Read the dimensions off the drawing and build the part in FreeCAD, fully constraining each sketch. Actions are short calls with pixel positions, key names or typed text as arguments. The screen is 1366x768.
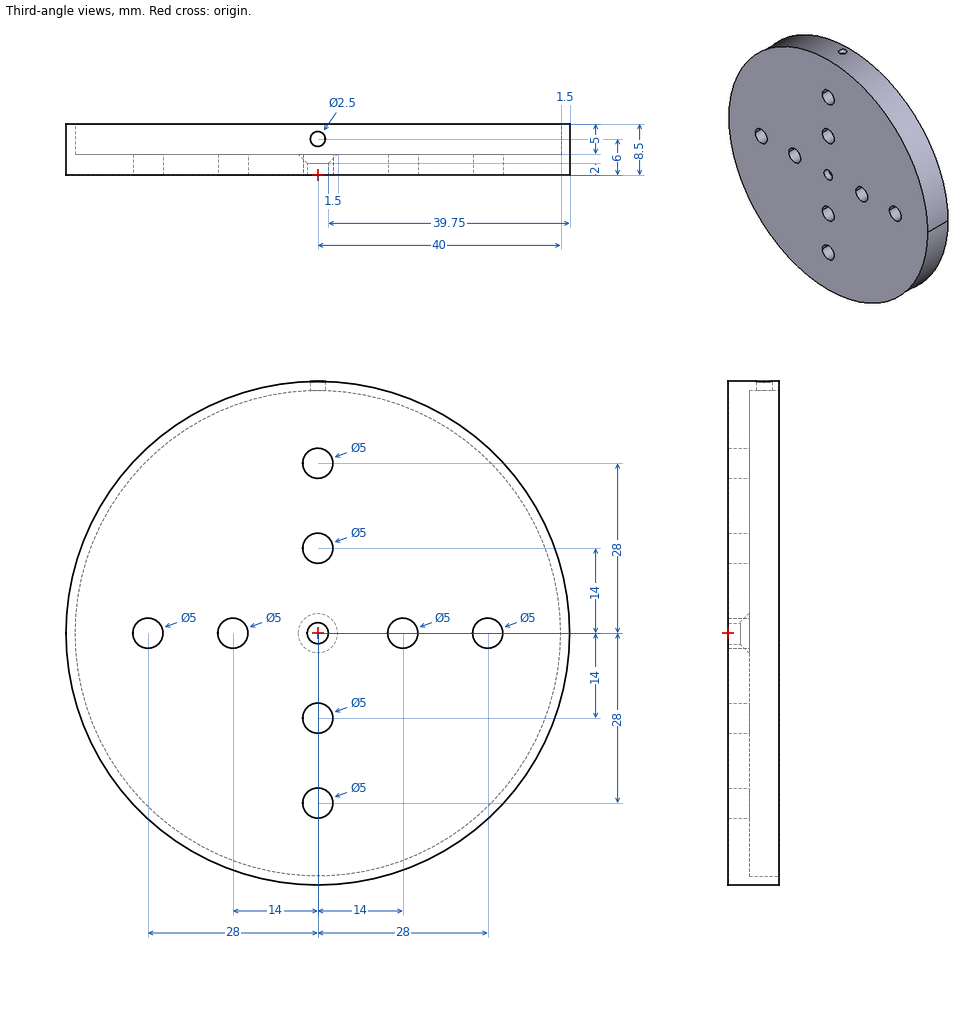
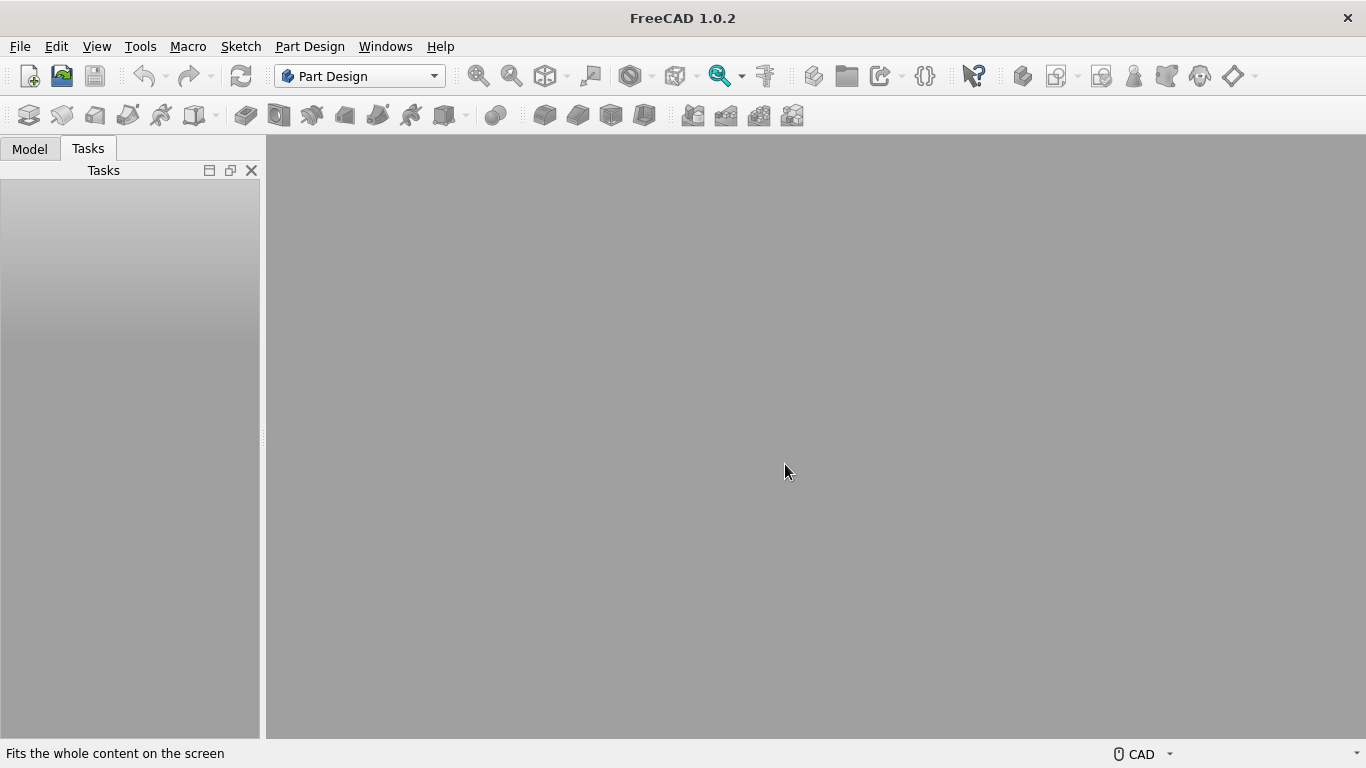
click(29, 76)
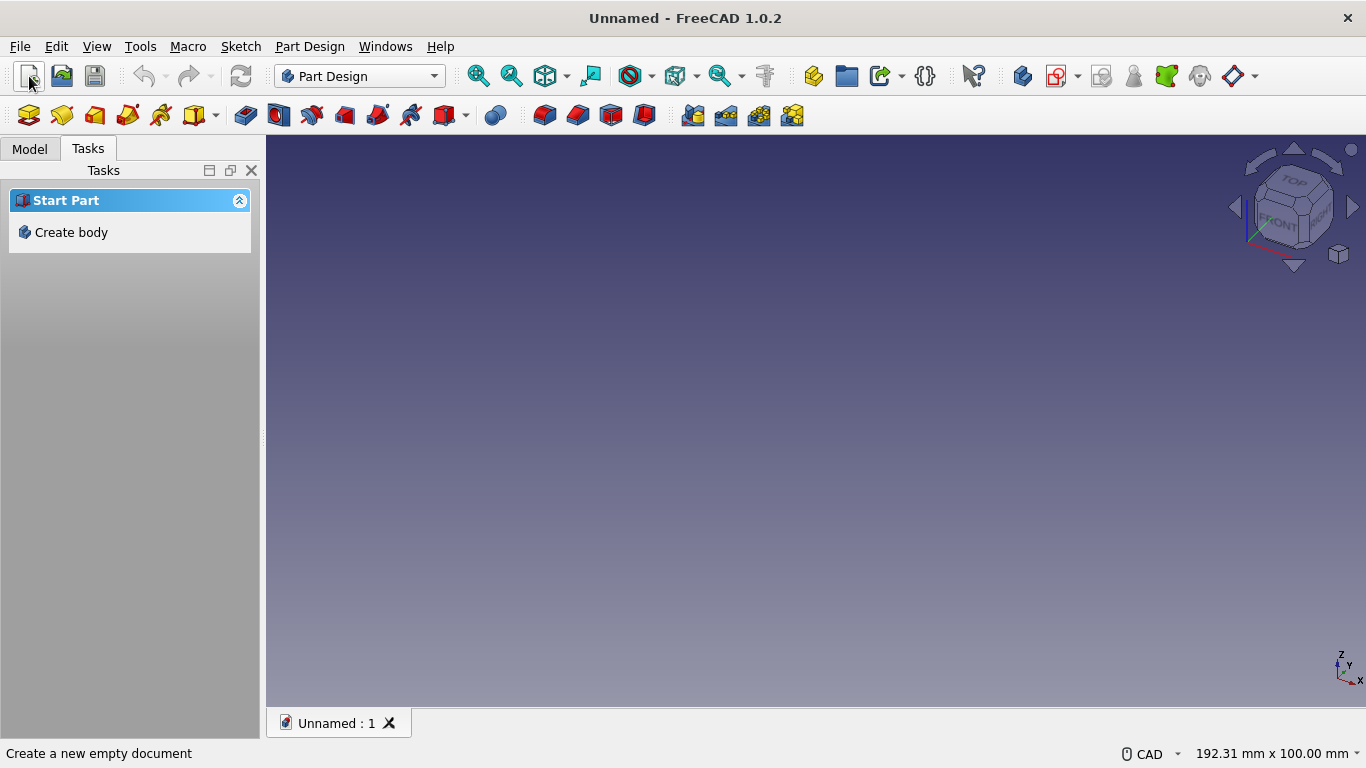
click(1056, 76)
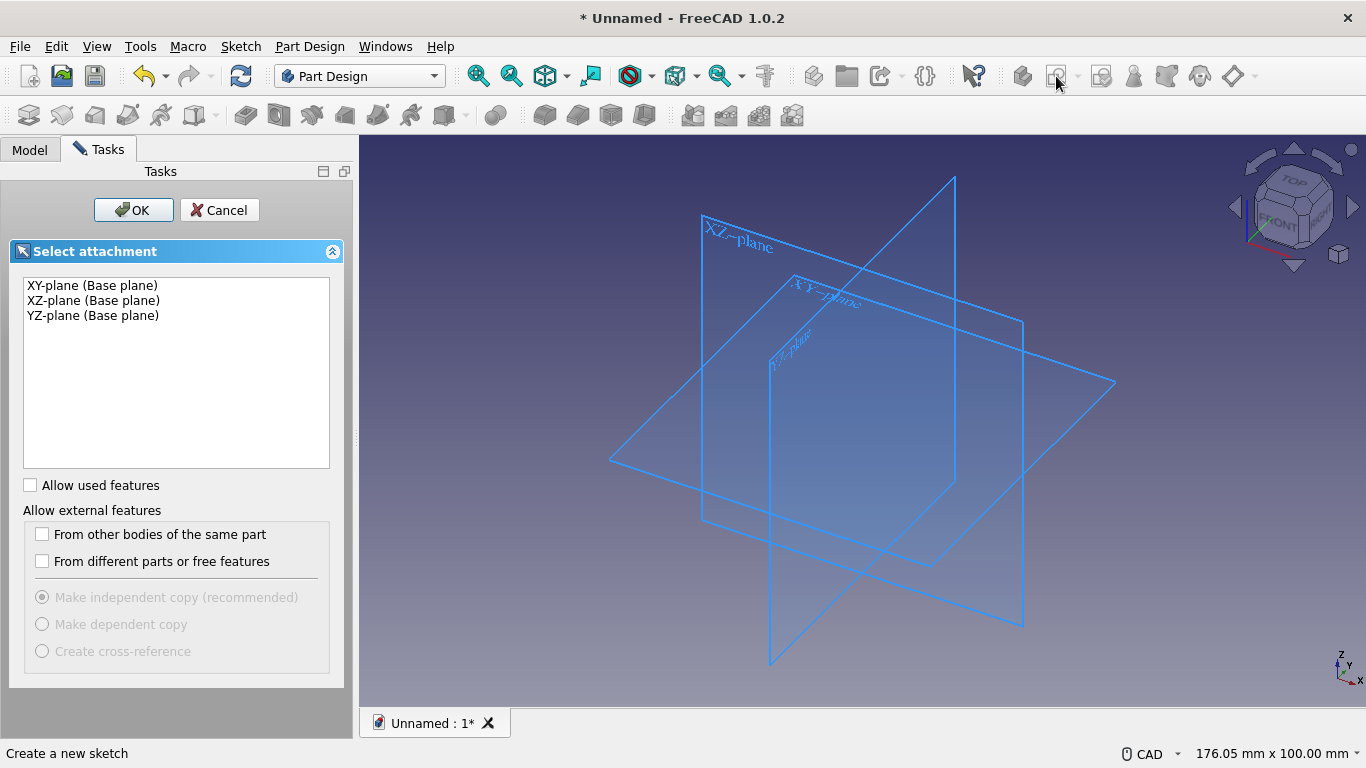
click(84, 286)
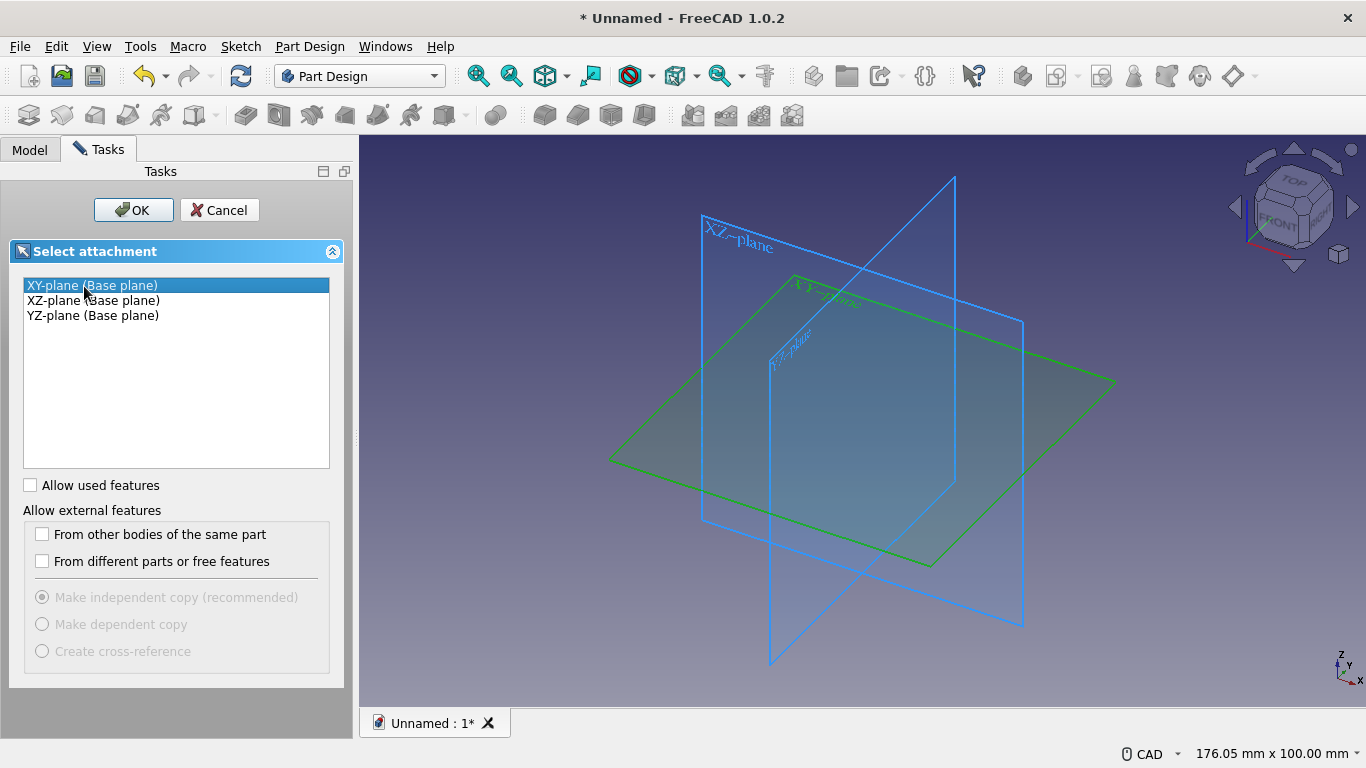
click(134, 210)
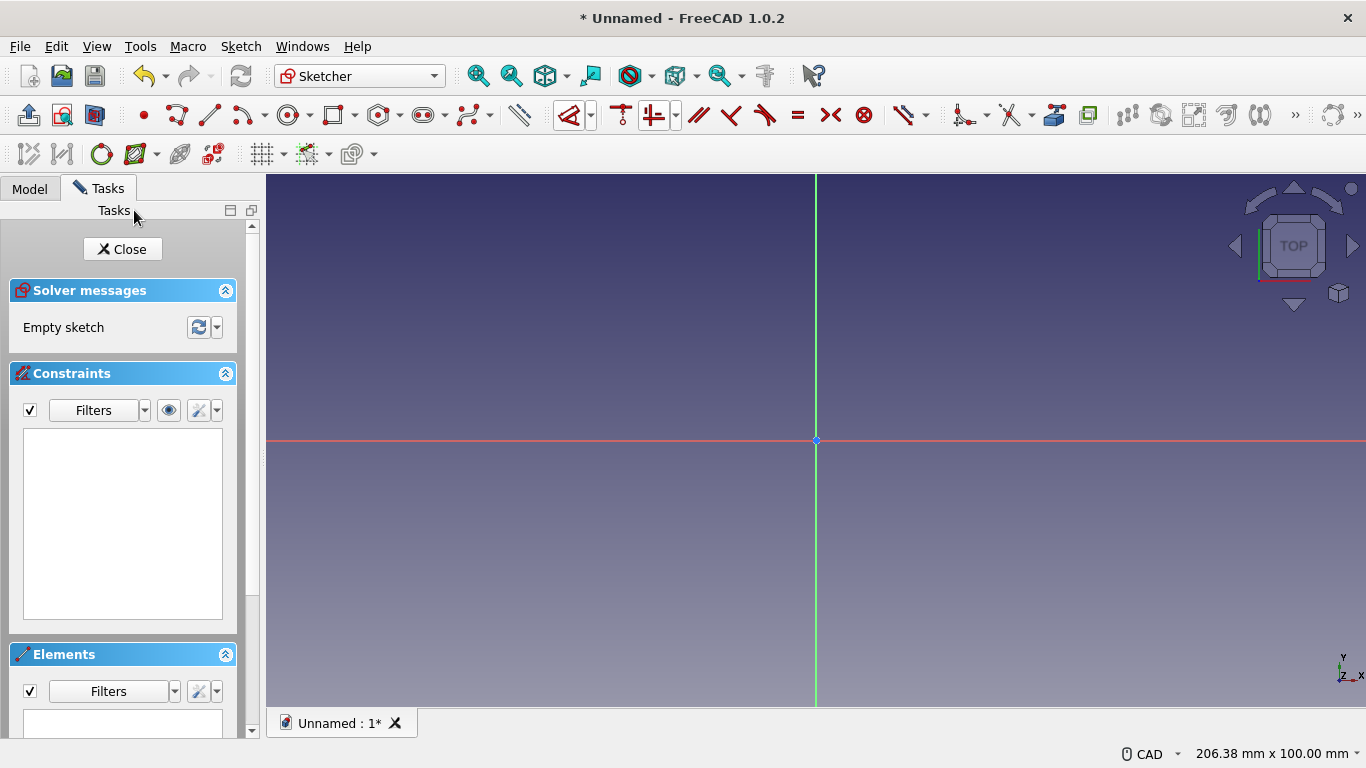
scroll(1031, 405, up, 5)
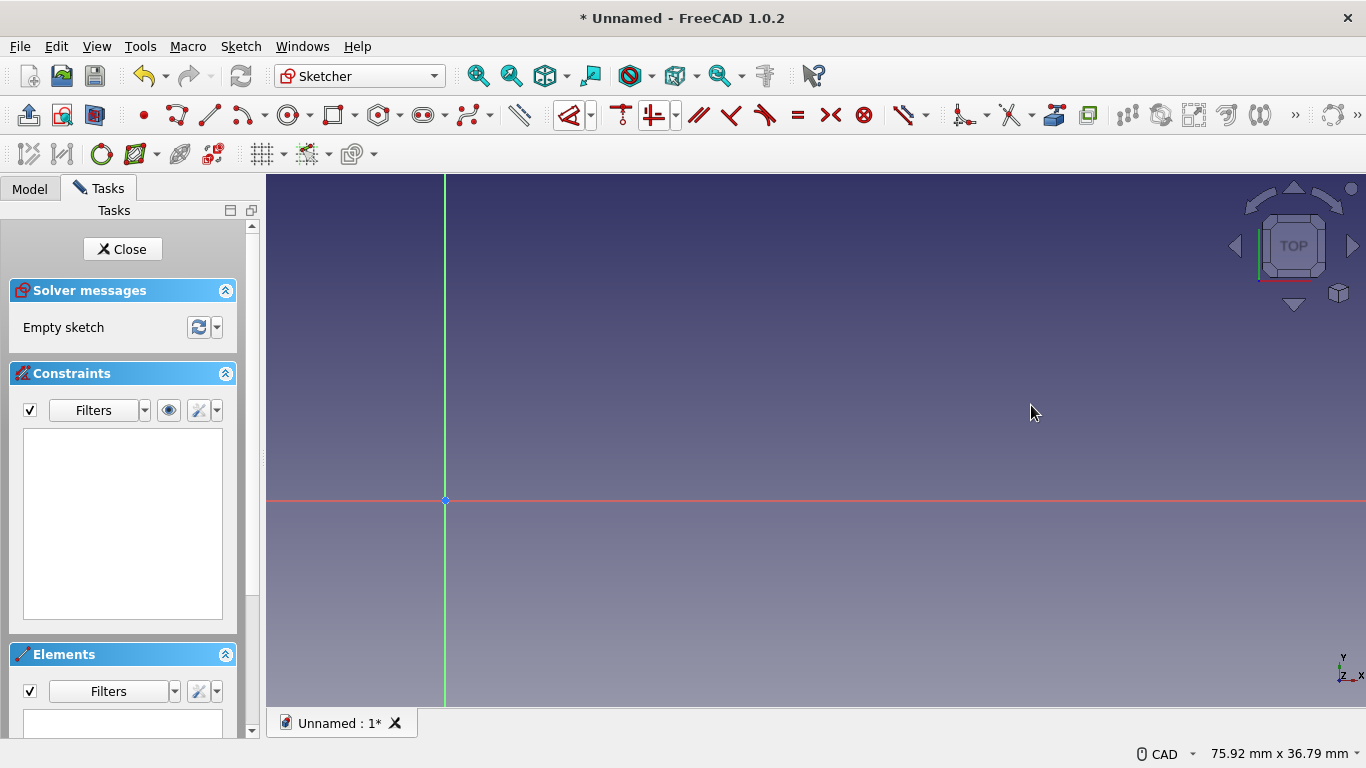
click(177, 116)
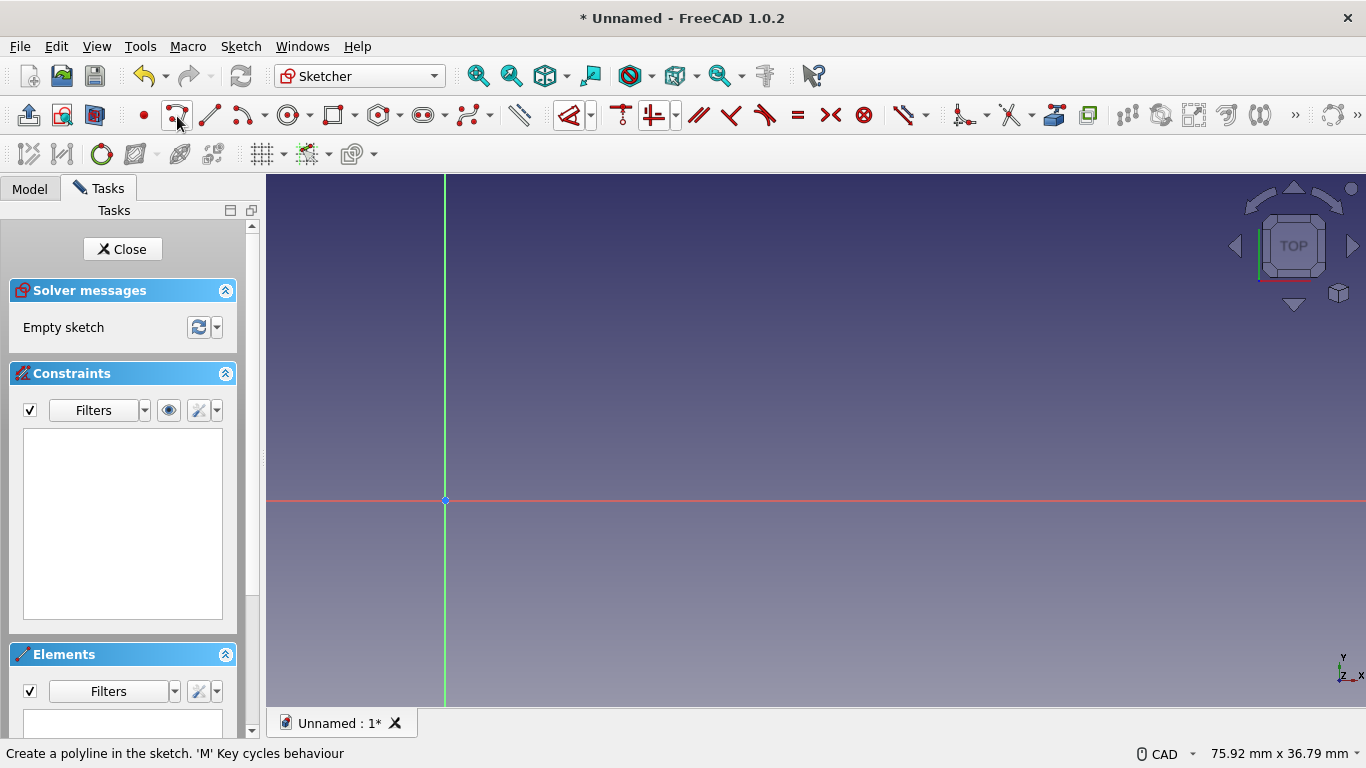
click(471, 501)
click(1047, 492)
click(1047, 378)
click(1025, 378)
click(1025, 450)
click(492, 450)
click(471, 472)
click(471, 501)
key(Escape)
key(Escape)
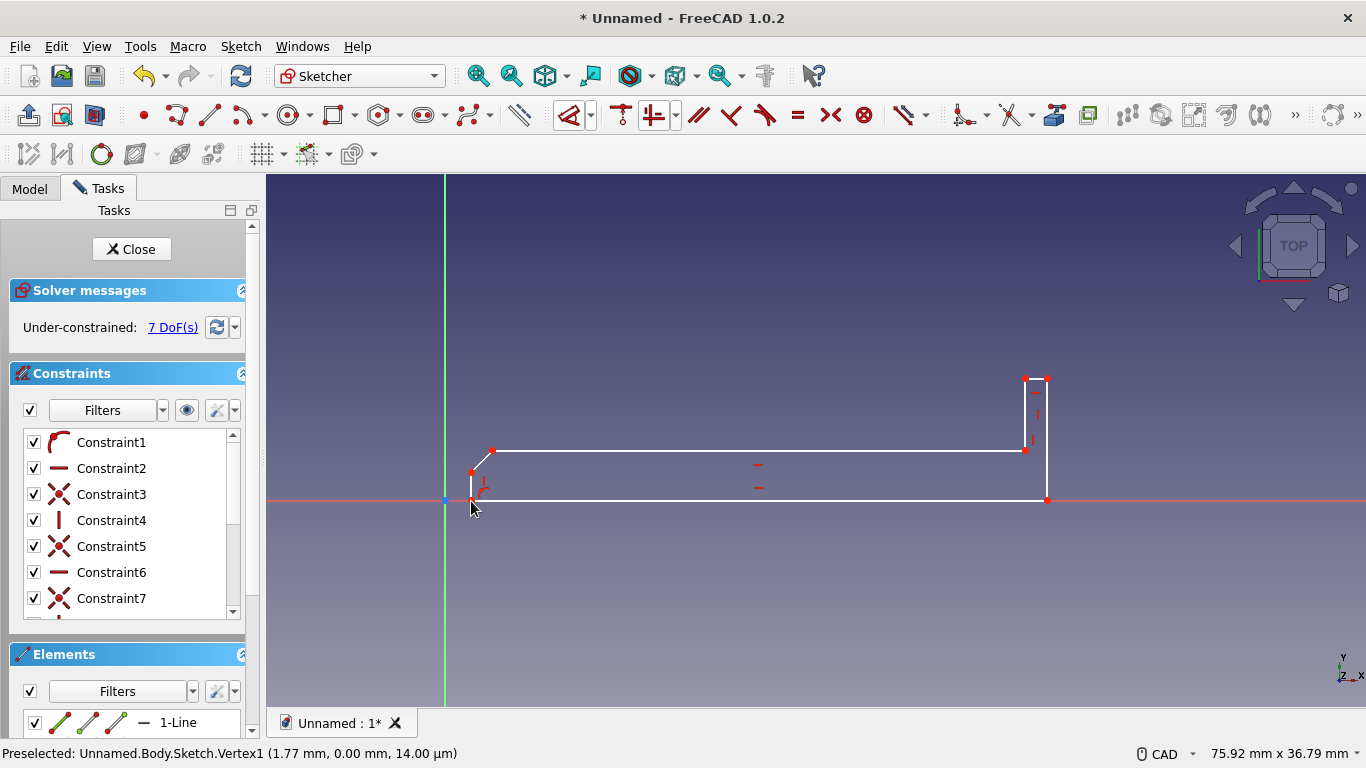
click(1025, 401)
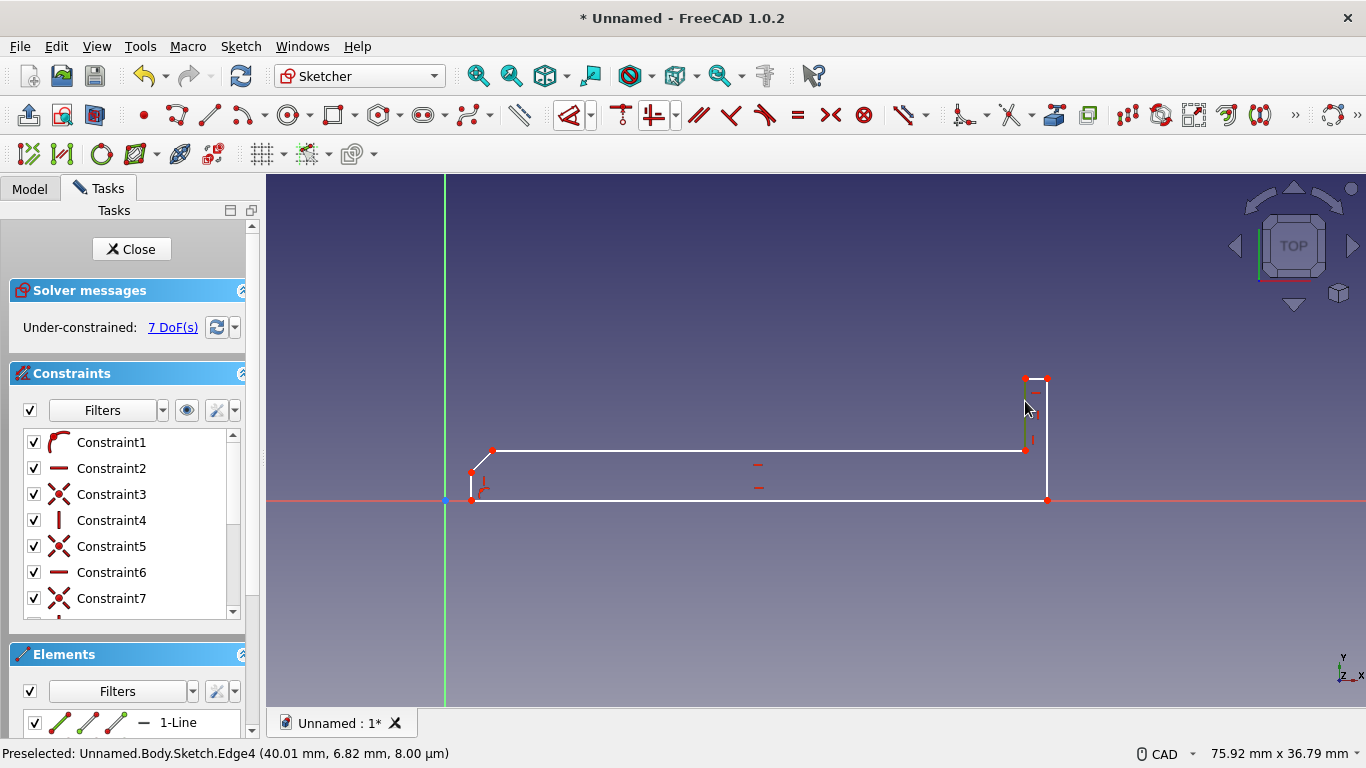
click(590, 116)